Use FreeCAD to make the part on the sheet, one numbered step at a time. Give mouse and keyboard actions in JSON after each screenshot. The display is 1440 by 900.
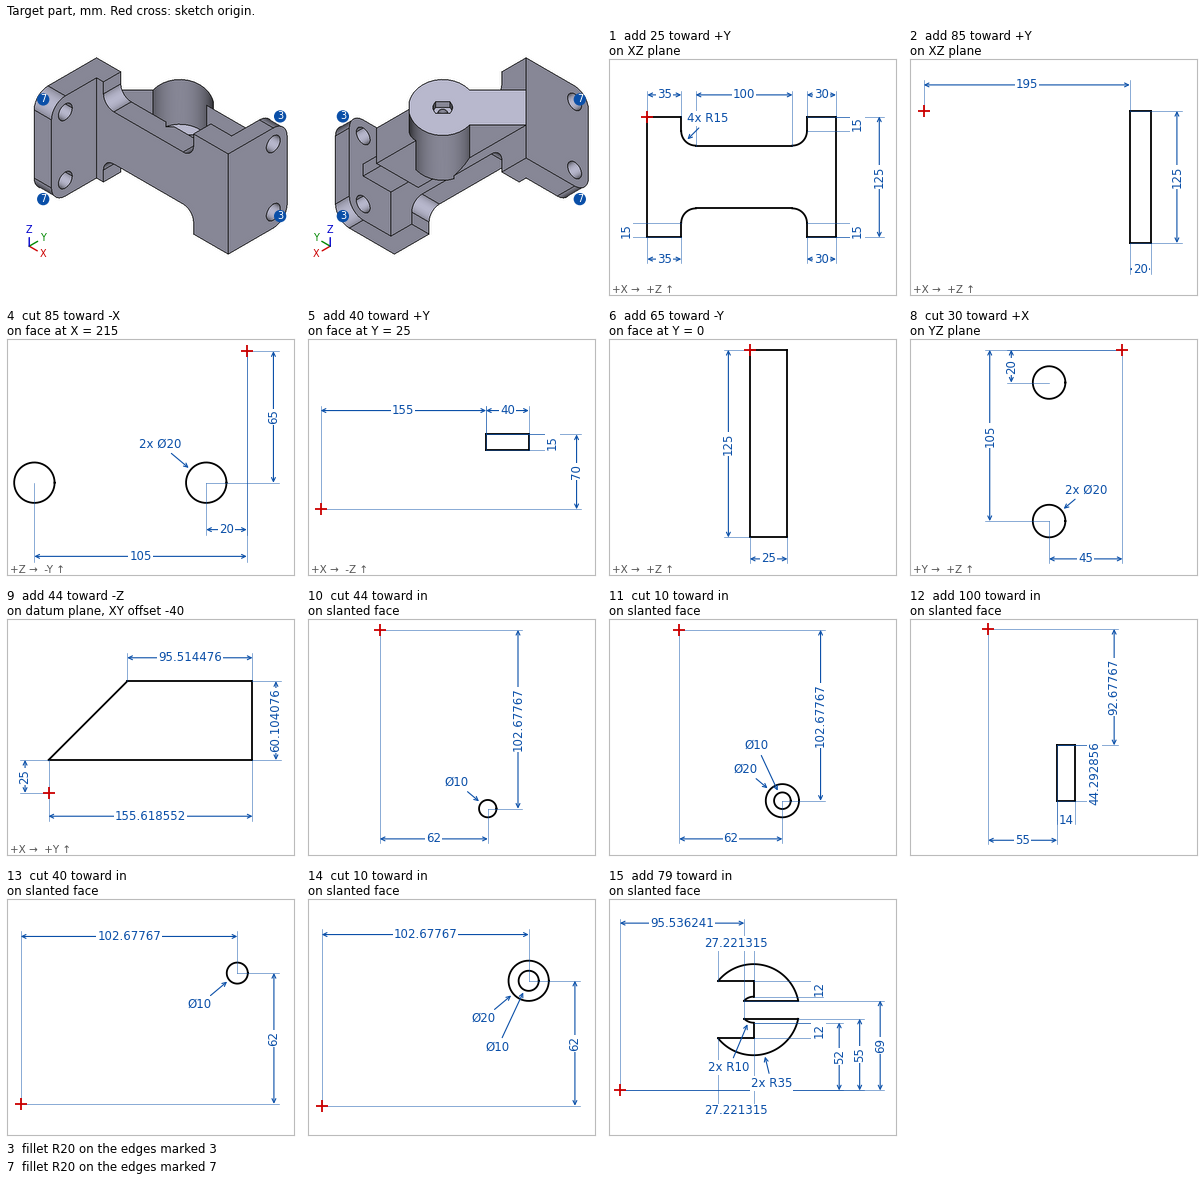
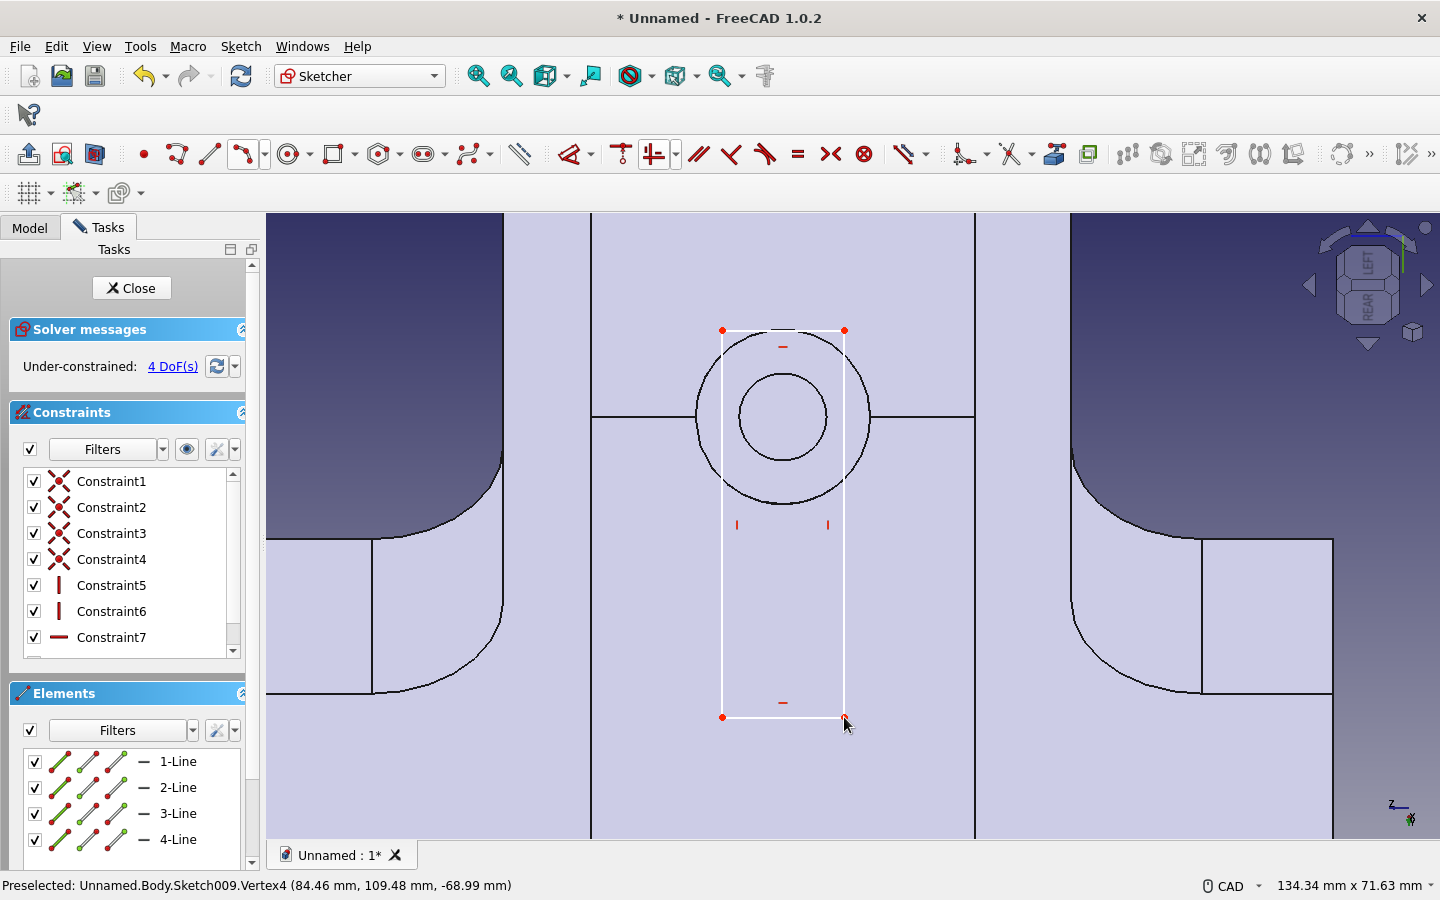
{"action": "left_click", "coordinate": [568, 154]}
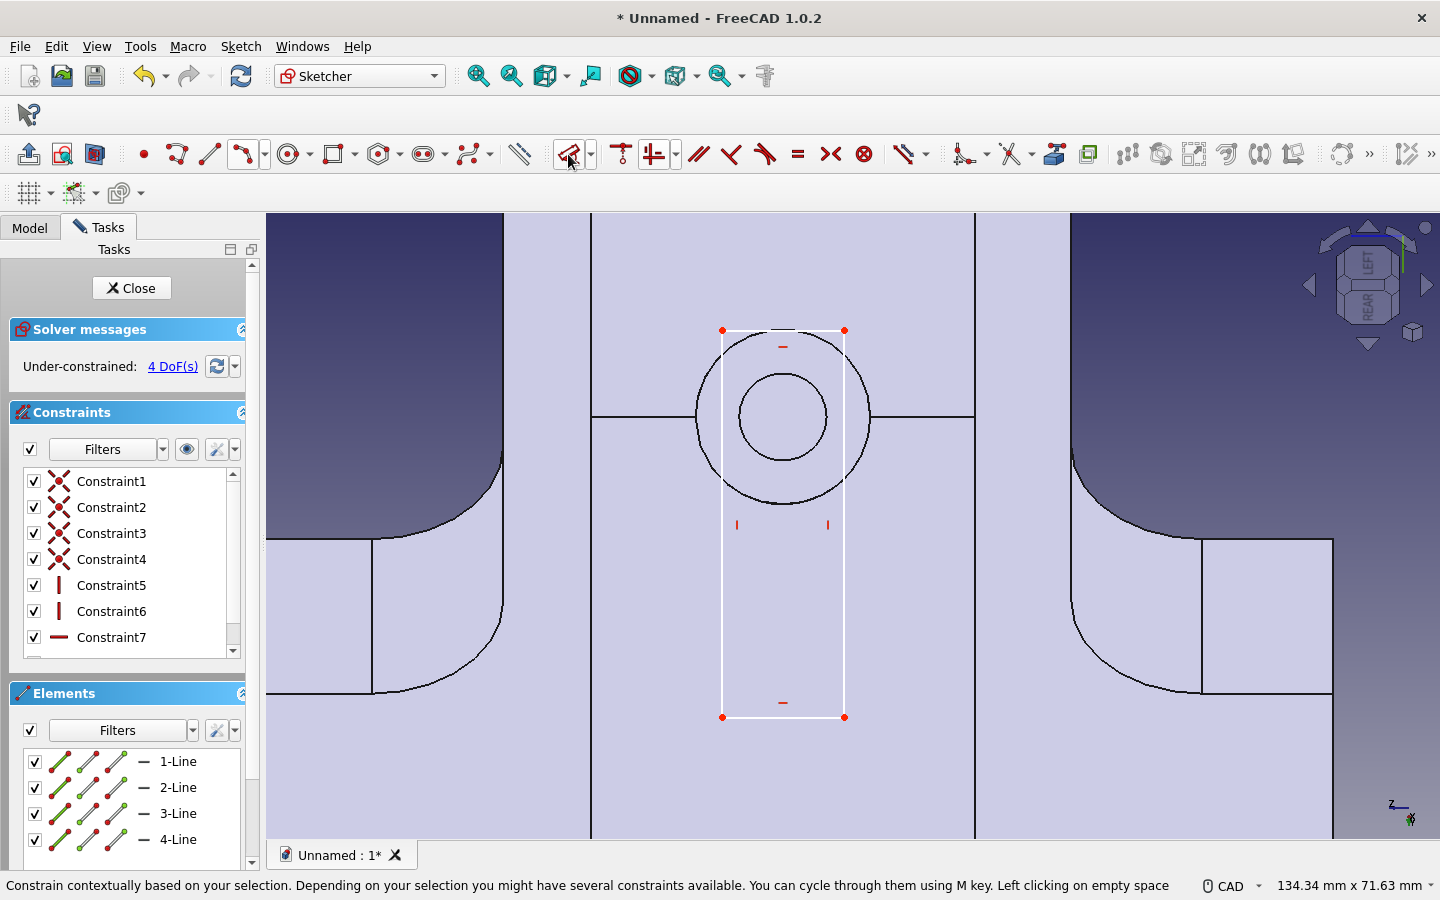
{"action": "left_click", "coordinate": [759, 718]}
{"action": "left_click", "coordinate": [783, 752]}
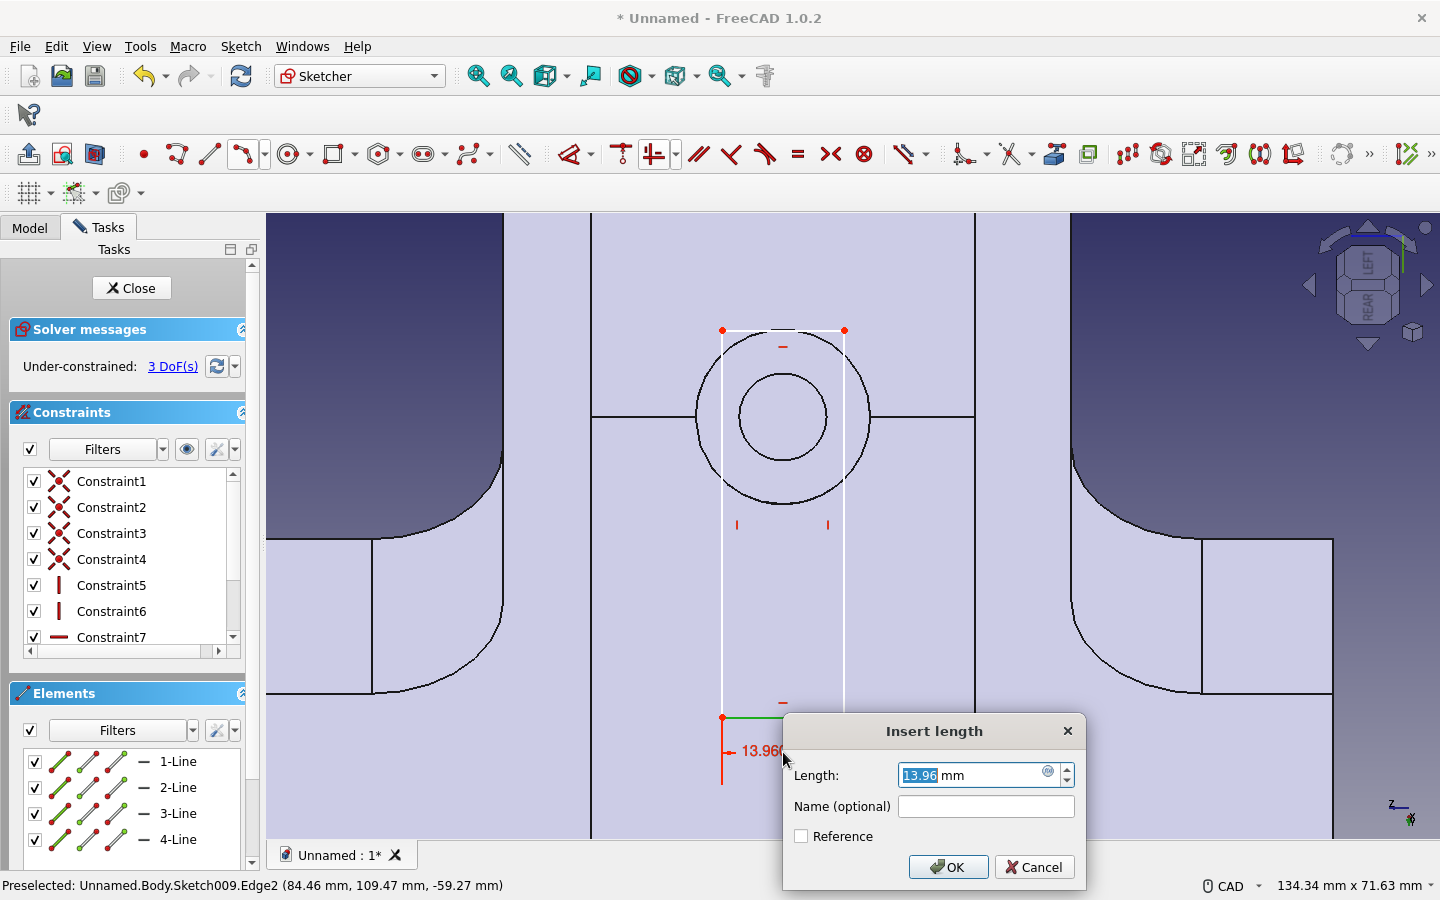
{"action": "type", "text": "14"}
{"action": "key", "text": "Return"}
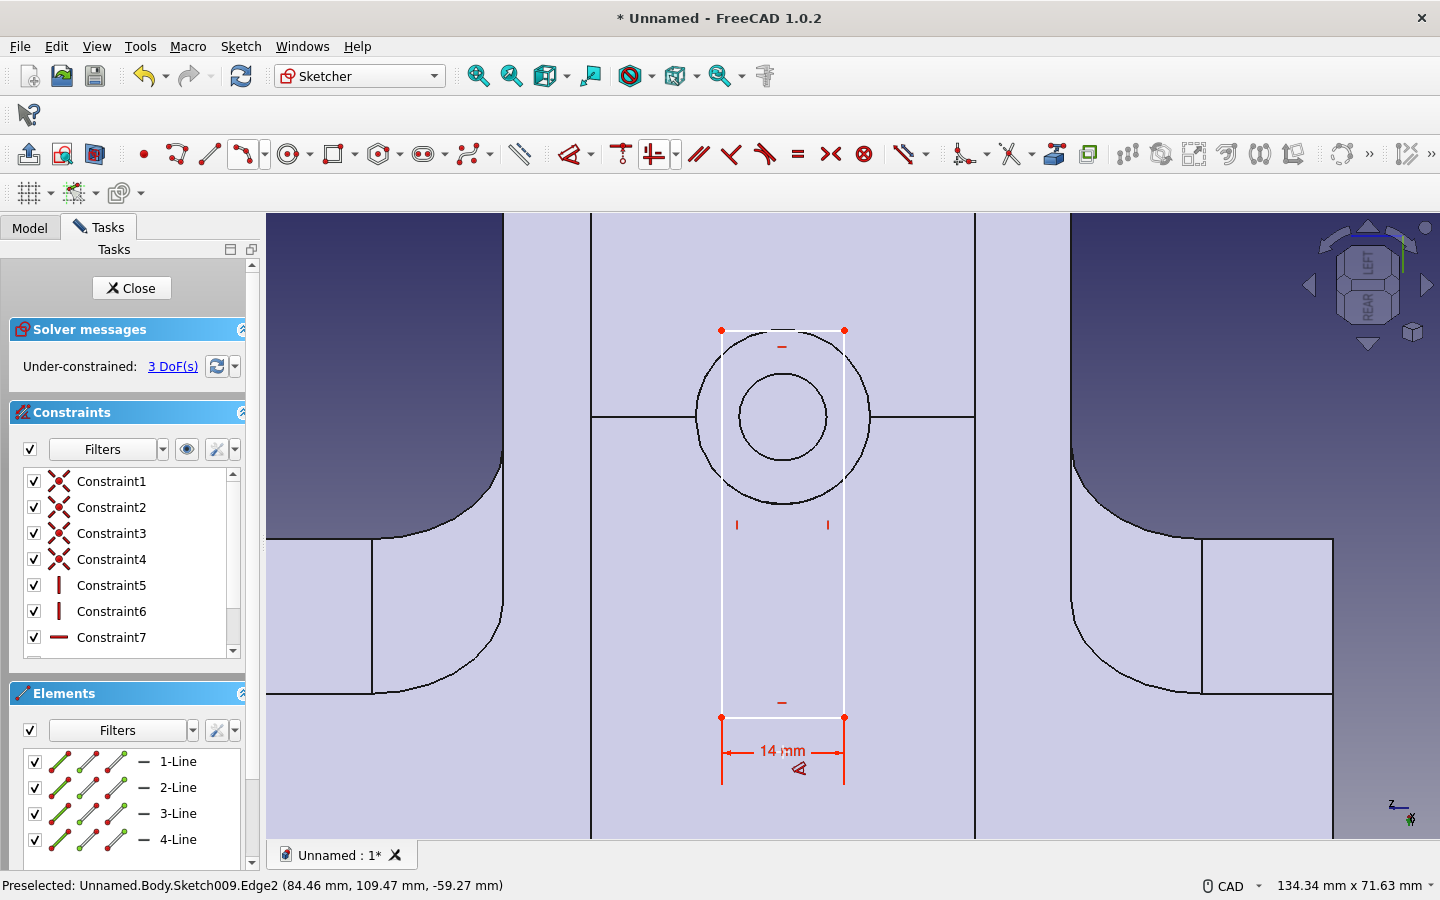
{"action": "left_click", "coordinate": [722, 331]}
{"action": "left_click", "coordinate": [508, 365]}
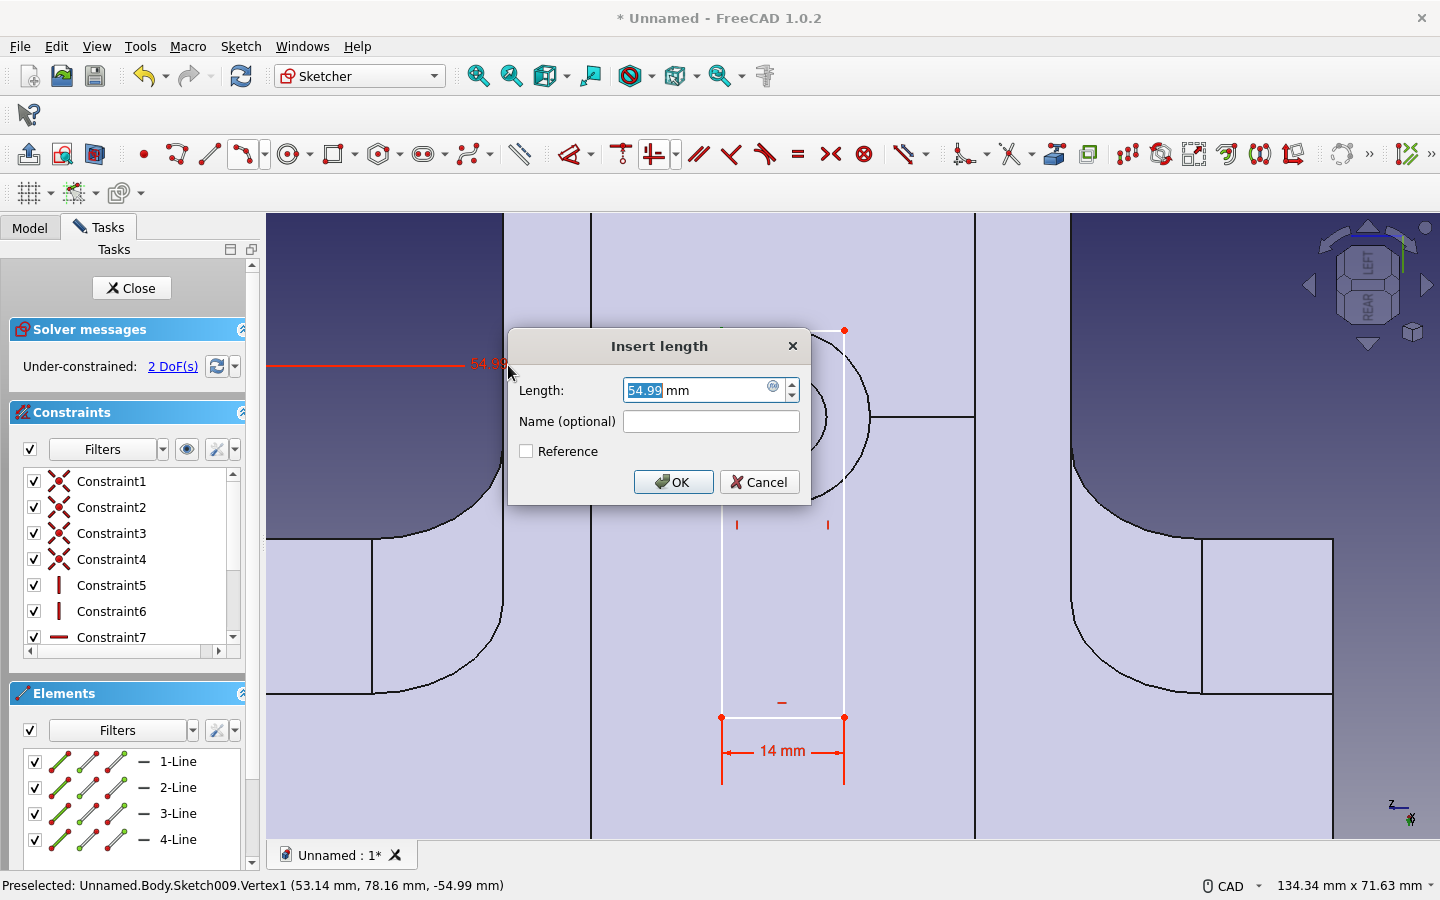
{"action": "type", "text": "55"}
{"action": "key", "text": "Return"}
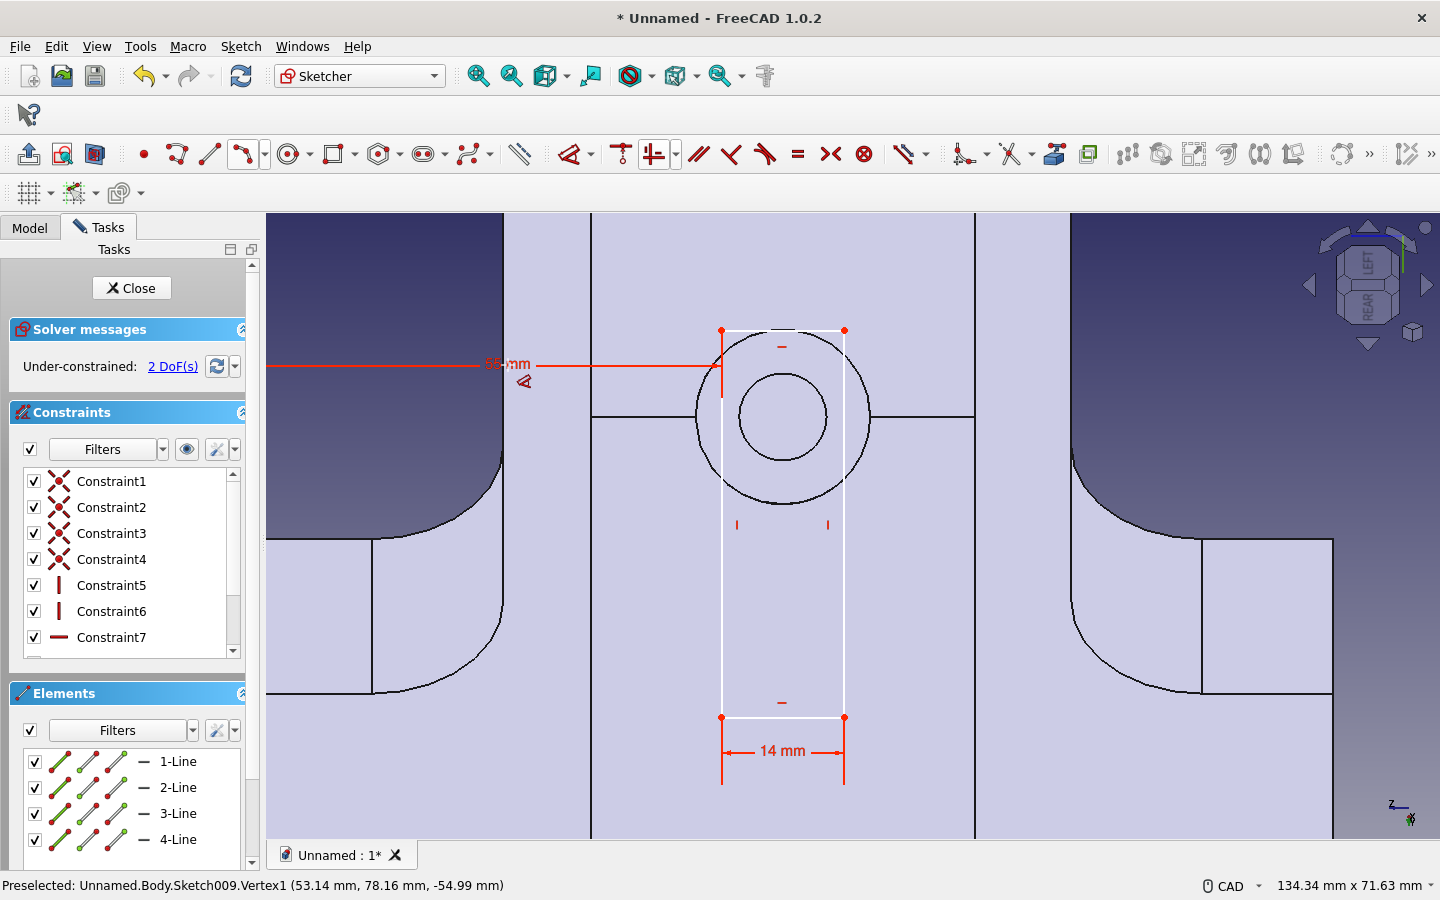
{"action": "left_click", "coordinate": [722, 447]}
{"action": "left_click", "coordinate": [688, 524]}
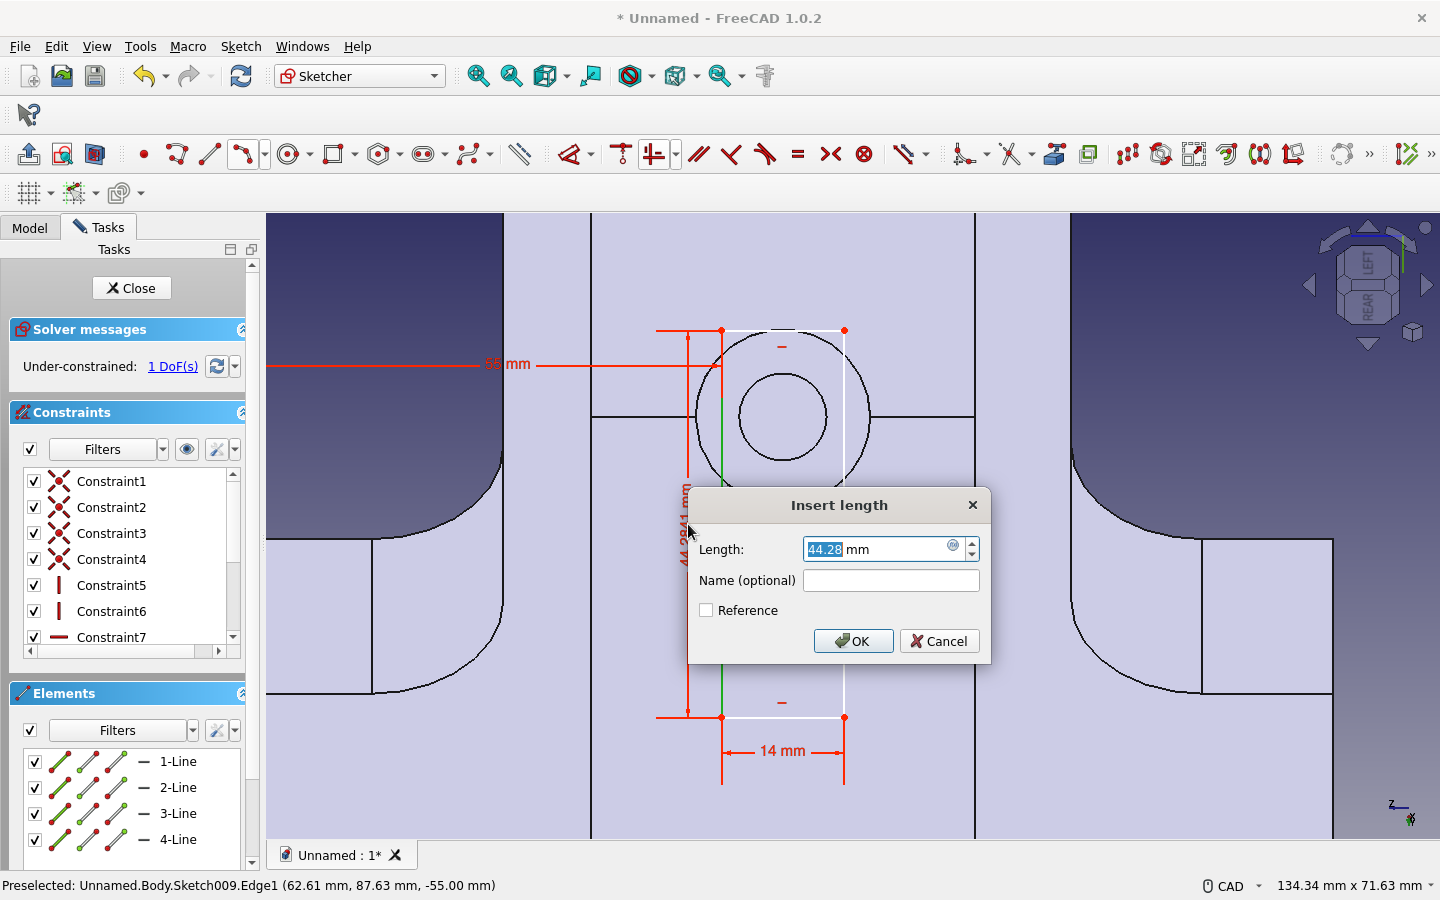
{"action": "type", "text": "44.292856"}
{"action": "key", "text": "Return"}